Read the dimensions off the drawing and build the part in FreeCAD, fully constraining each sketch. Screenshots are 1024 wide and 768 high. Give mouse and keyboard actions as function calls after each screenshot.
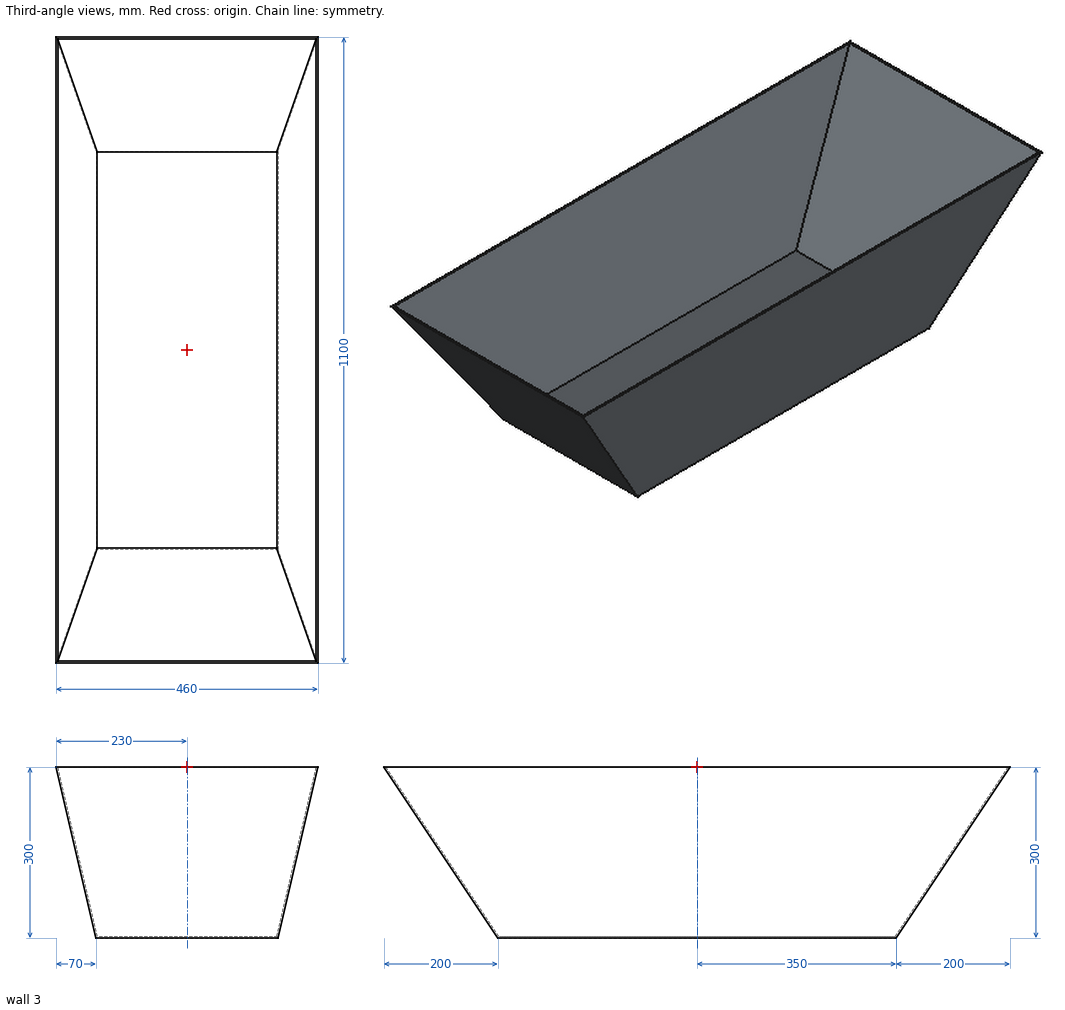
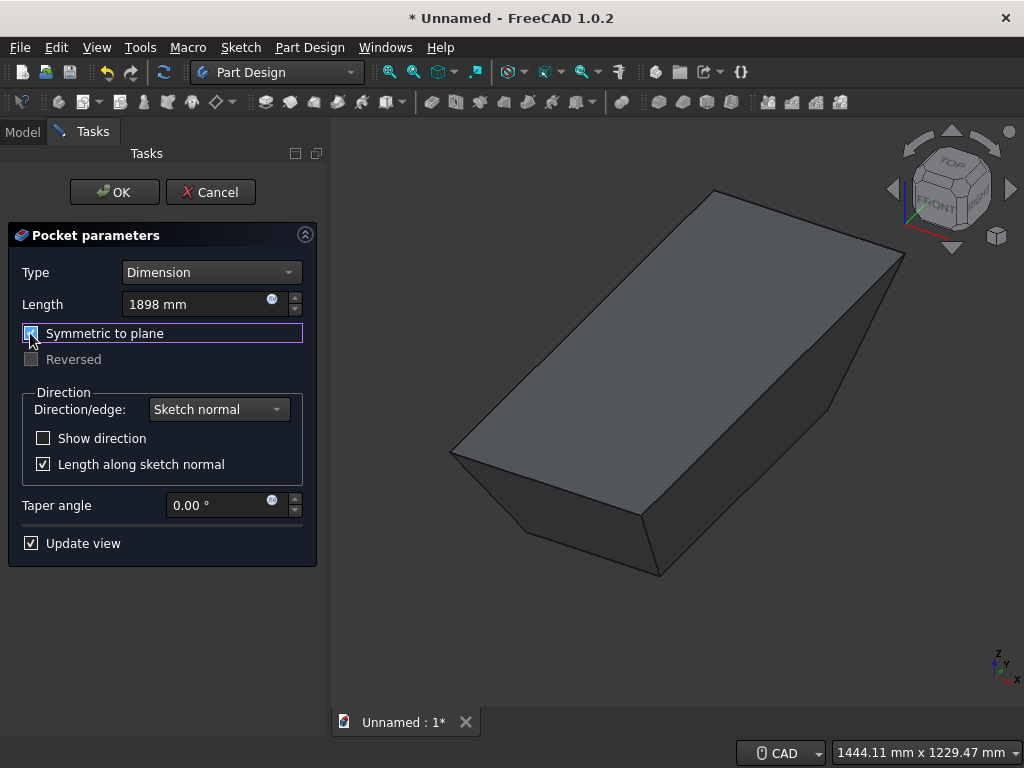
click(115, 192)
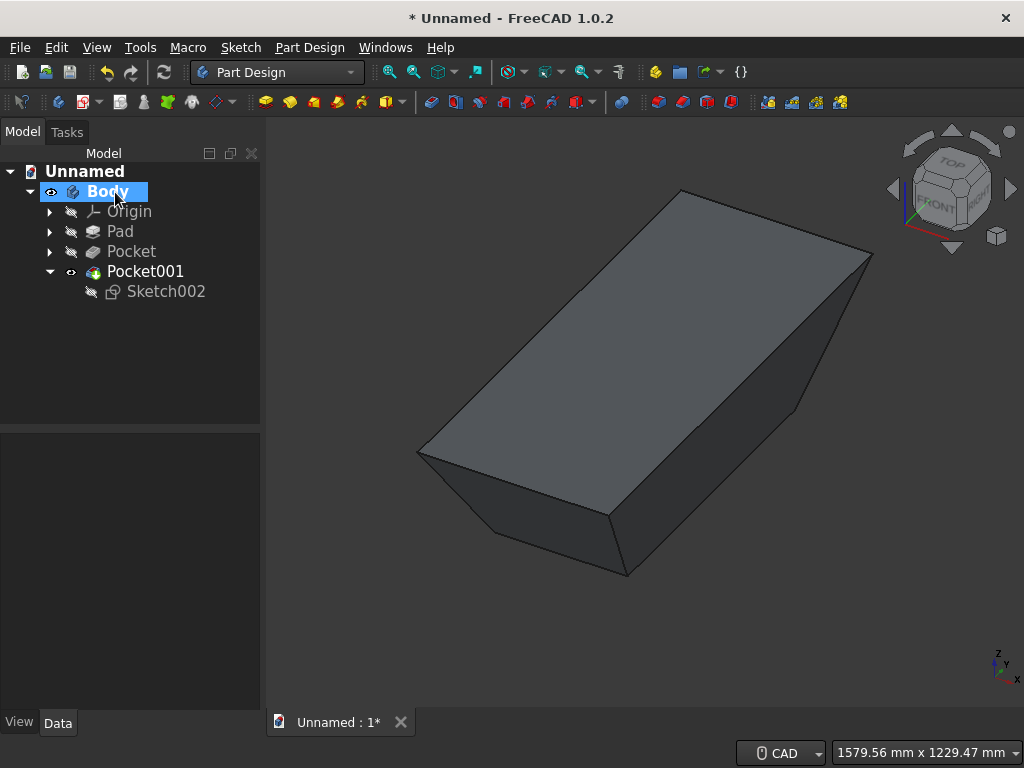
click(720, 277)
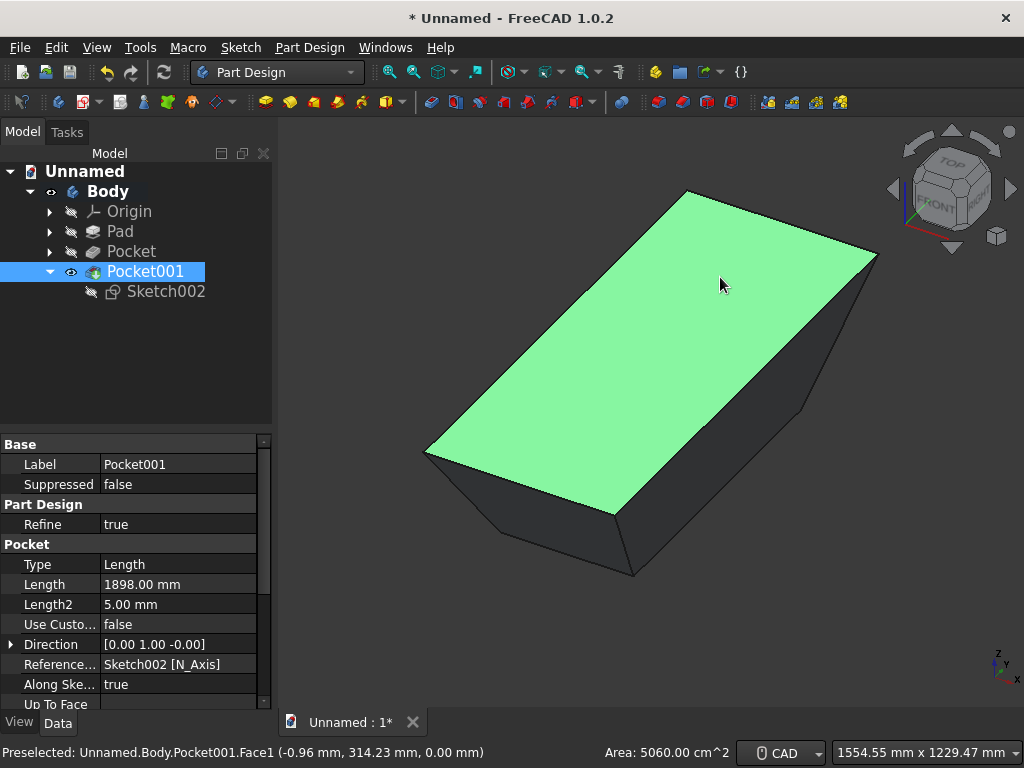
click(732, 102)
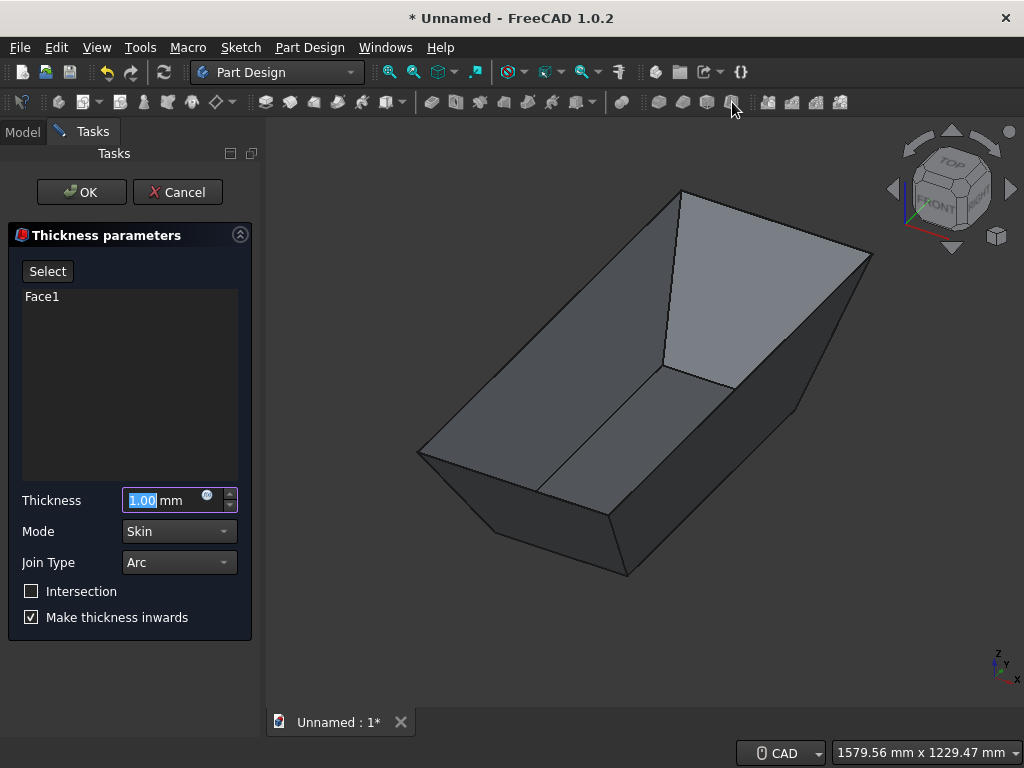
text(3)
key(Tab)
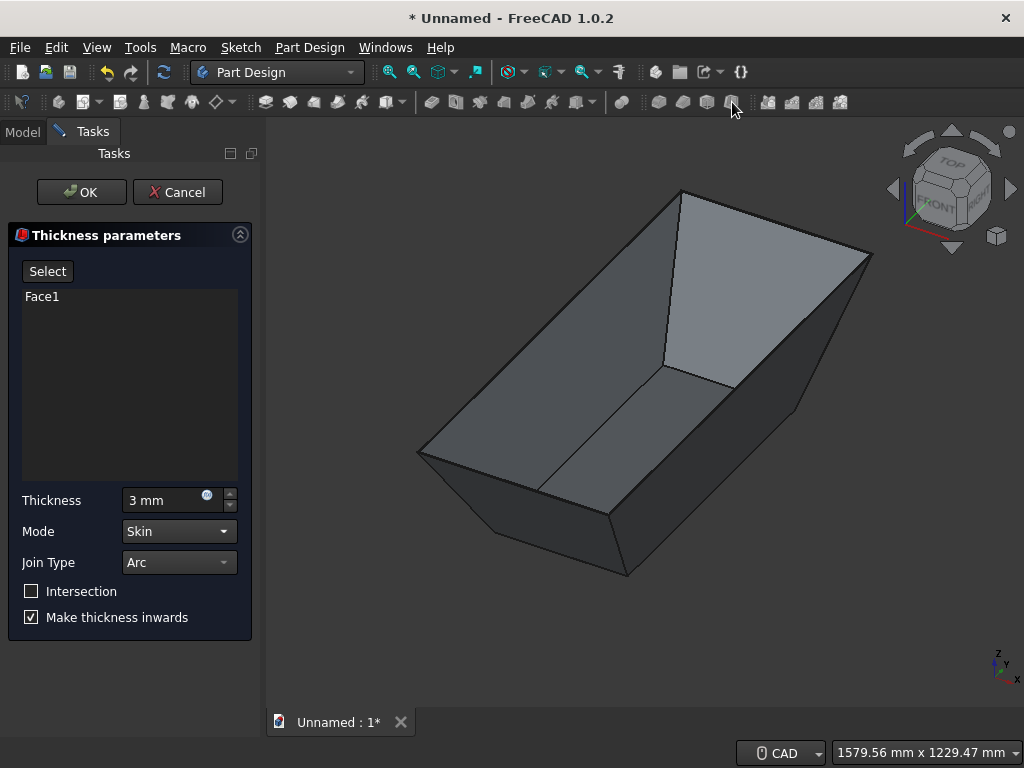
click(180, 562)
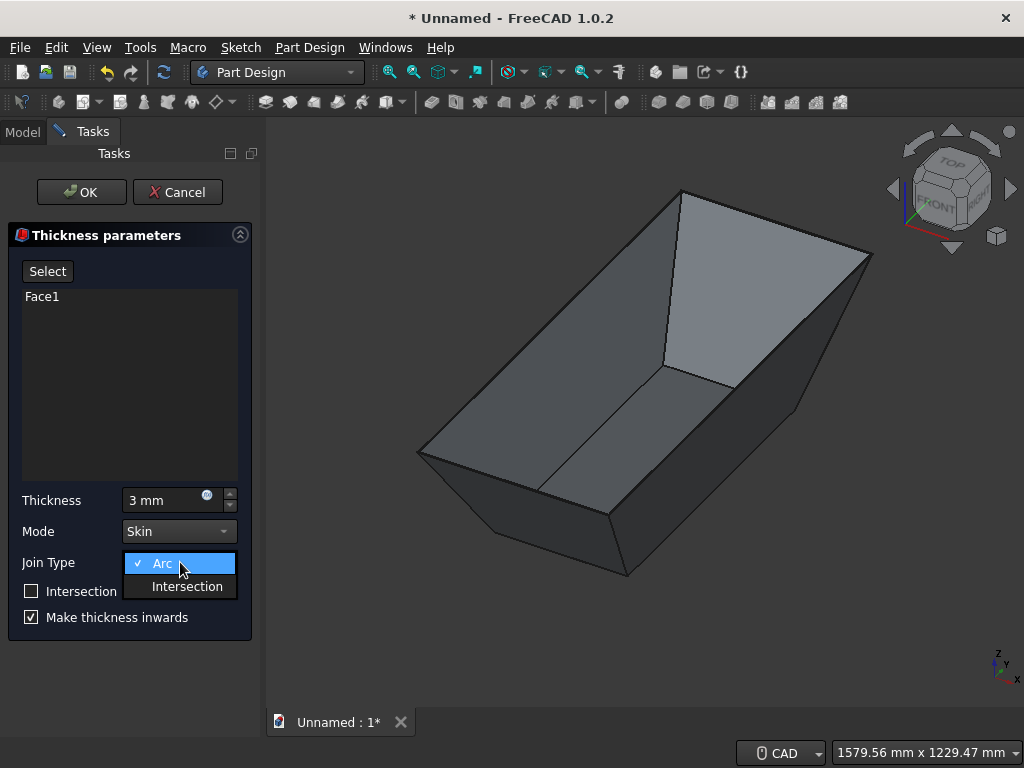
click(179, 586)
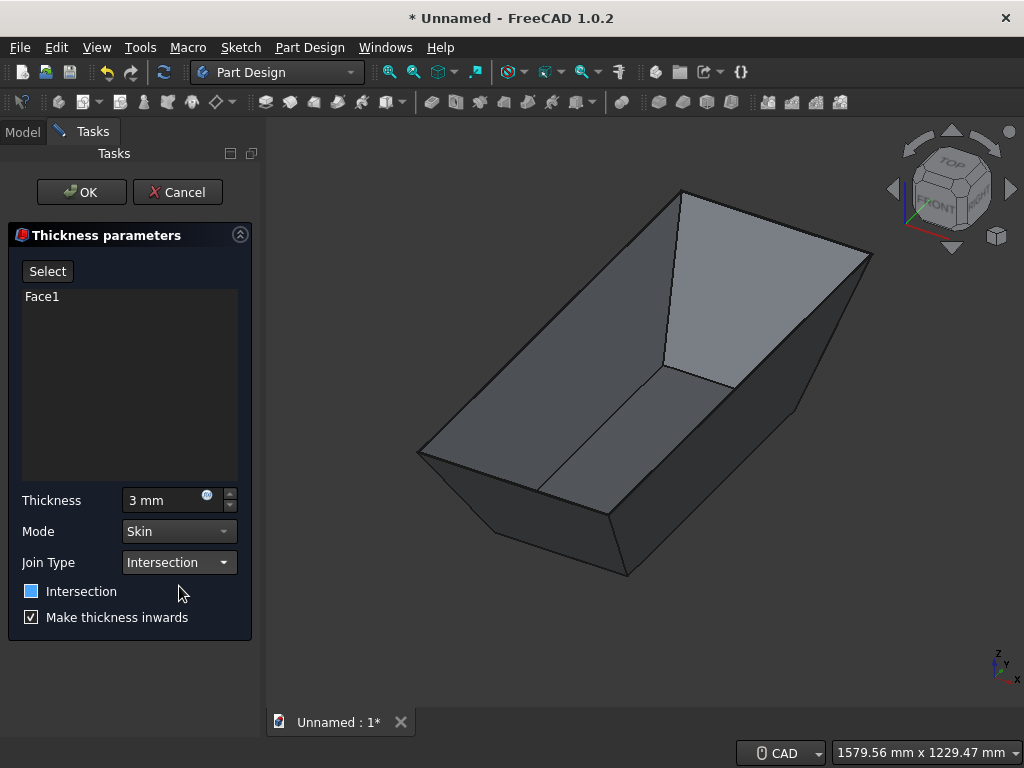
click(82, 192)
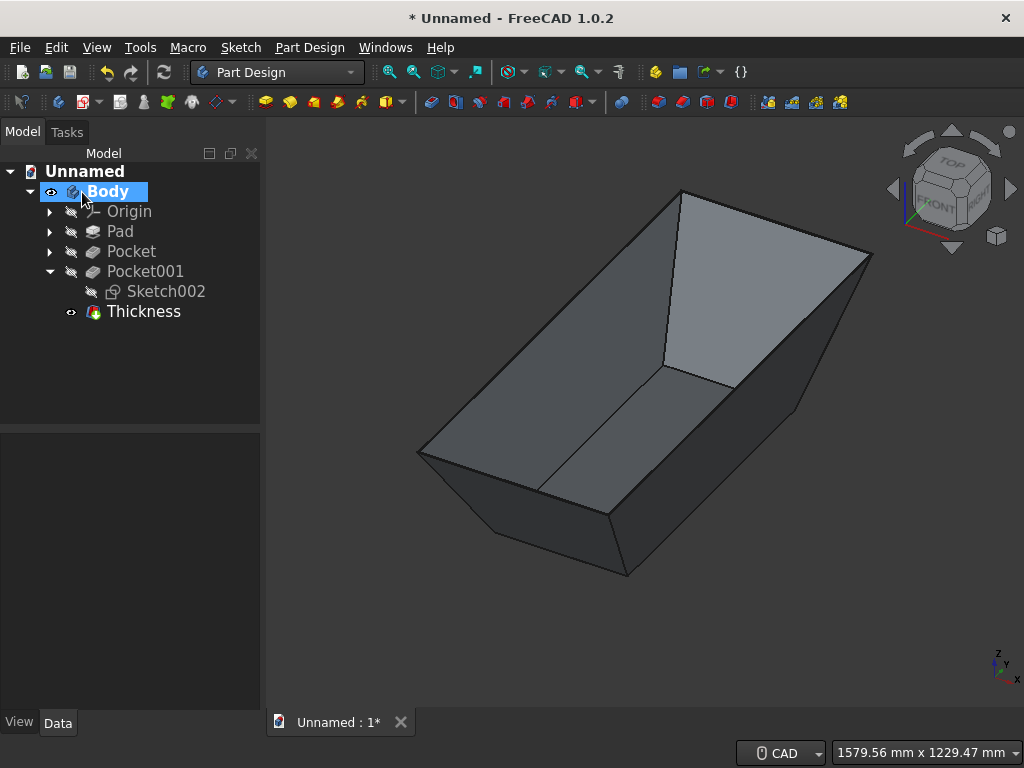
key(0)